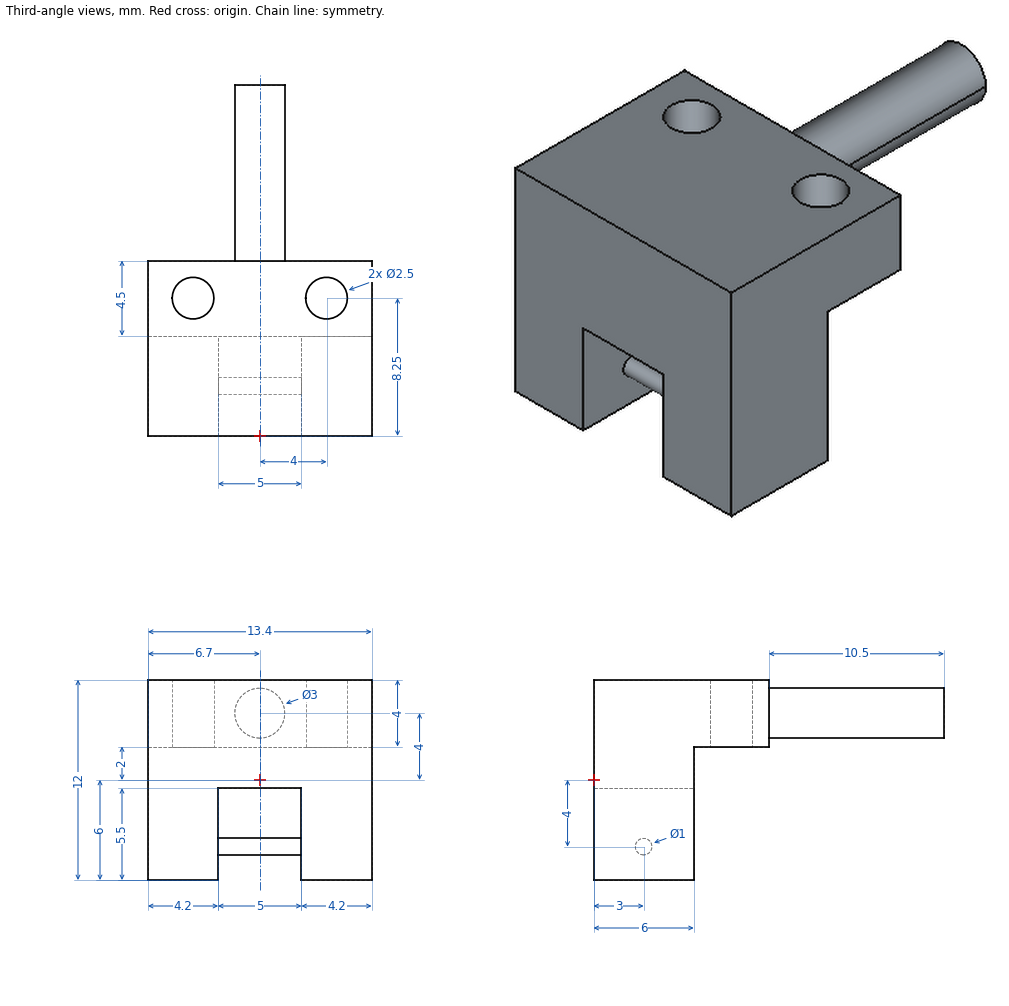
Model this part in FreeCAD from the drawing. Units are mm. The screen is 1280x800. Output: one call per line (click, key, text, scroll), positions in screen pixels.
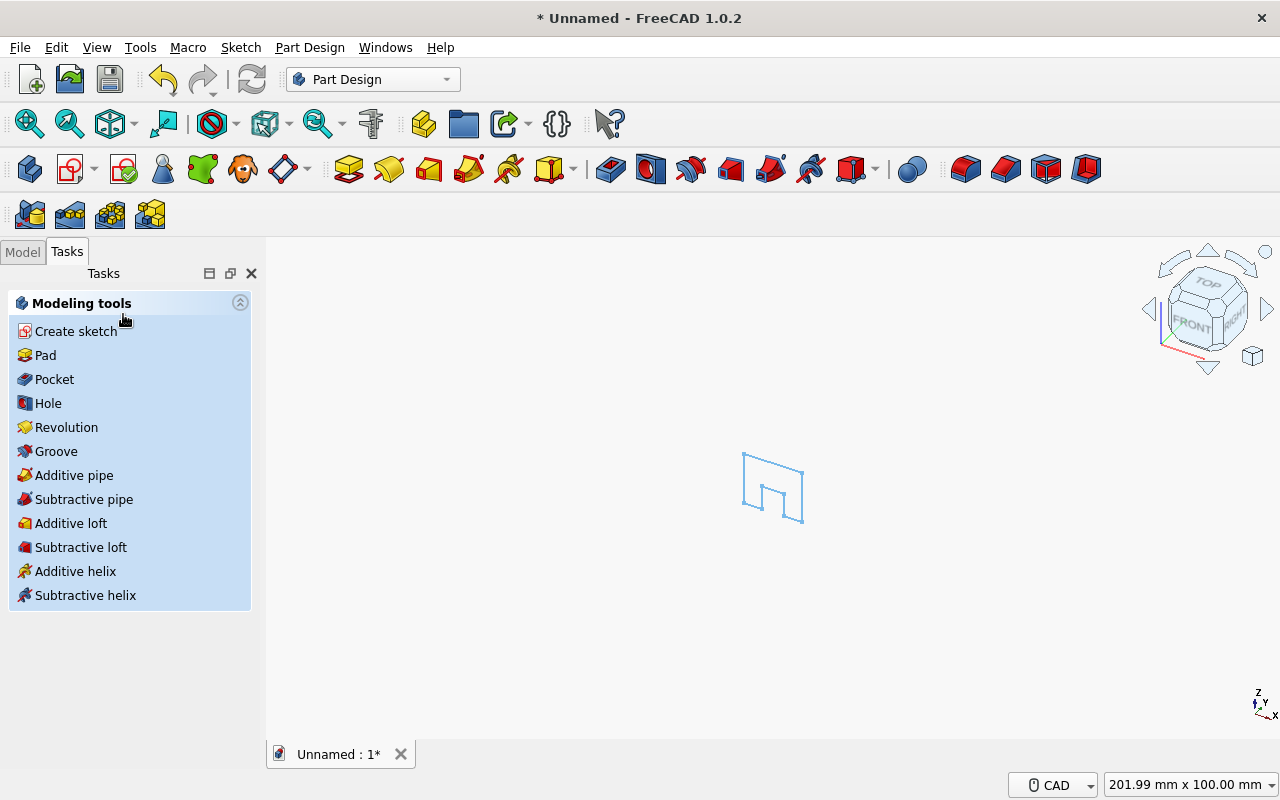
click(350, 170)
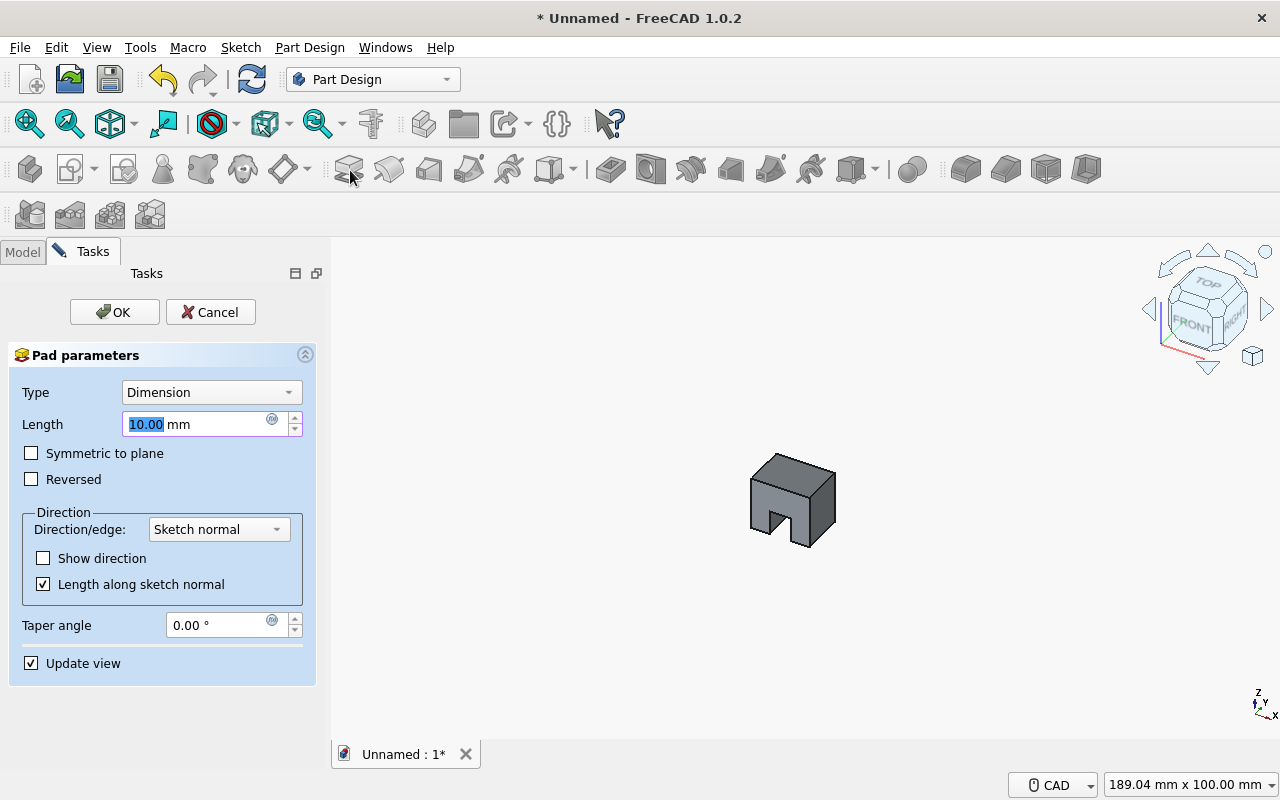
text(6)
key(Tab)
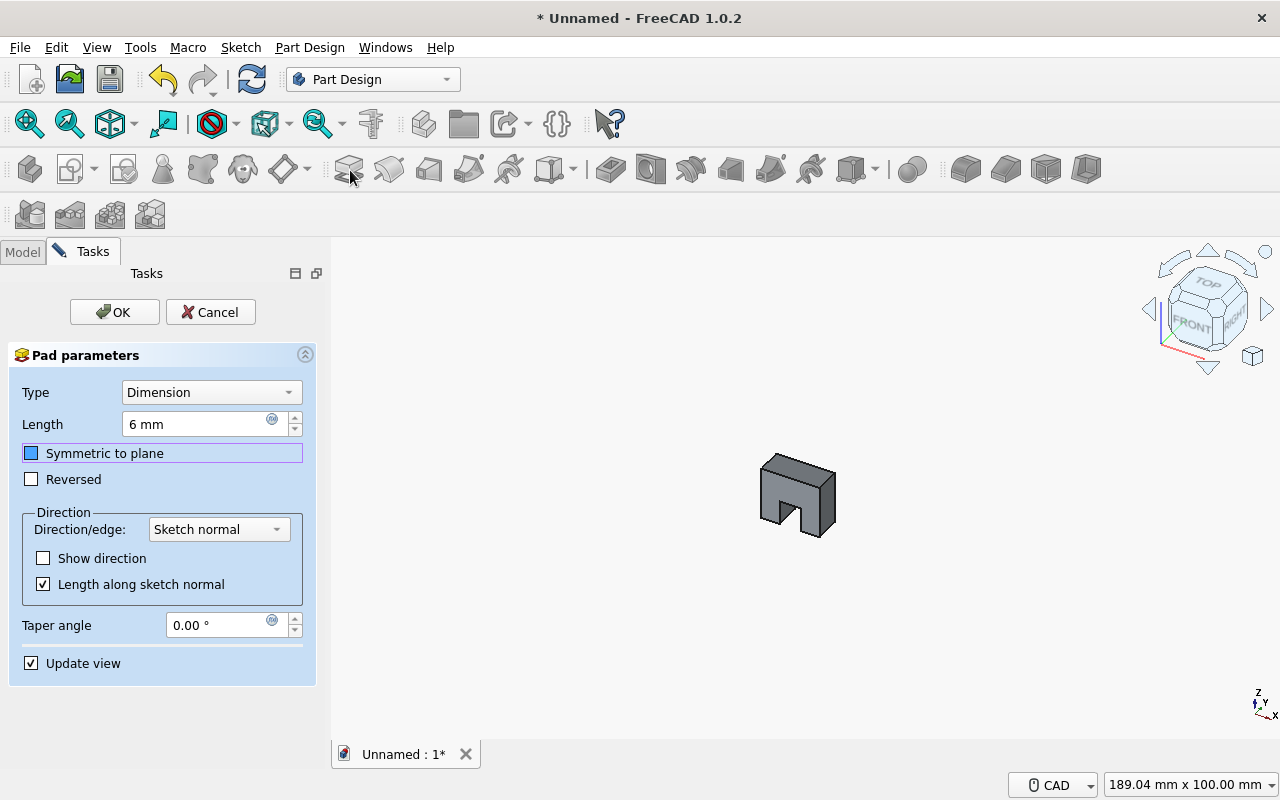
click(30, 479)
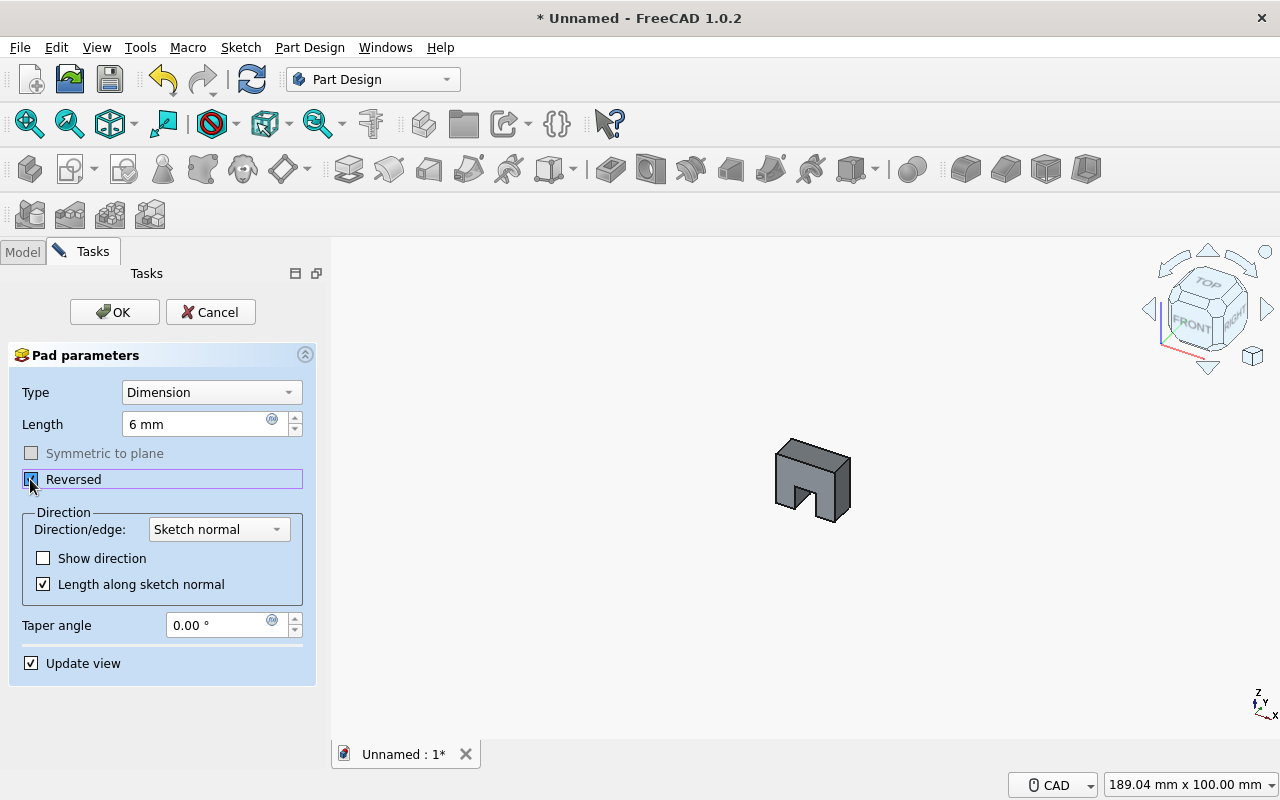
click(115, 312)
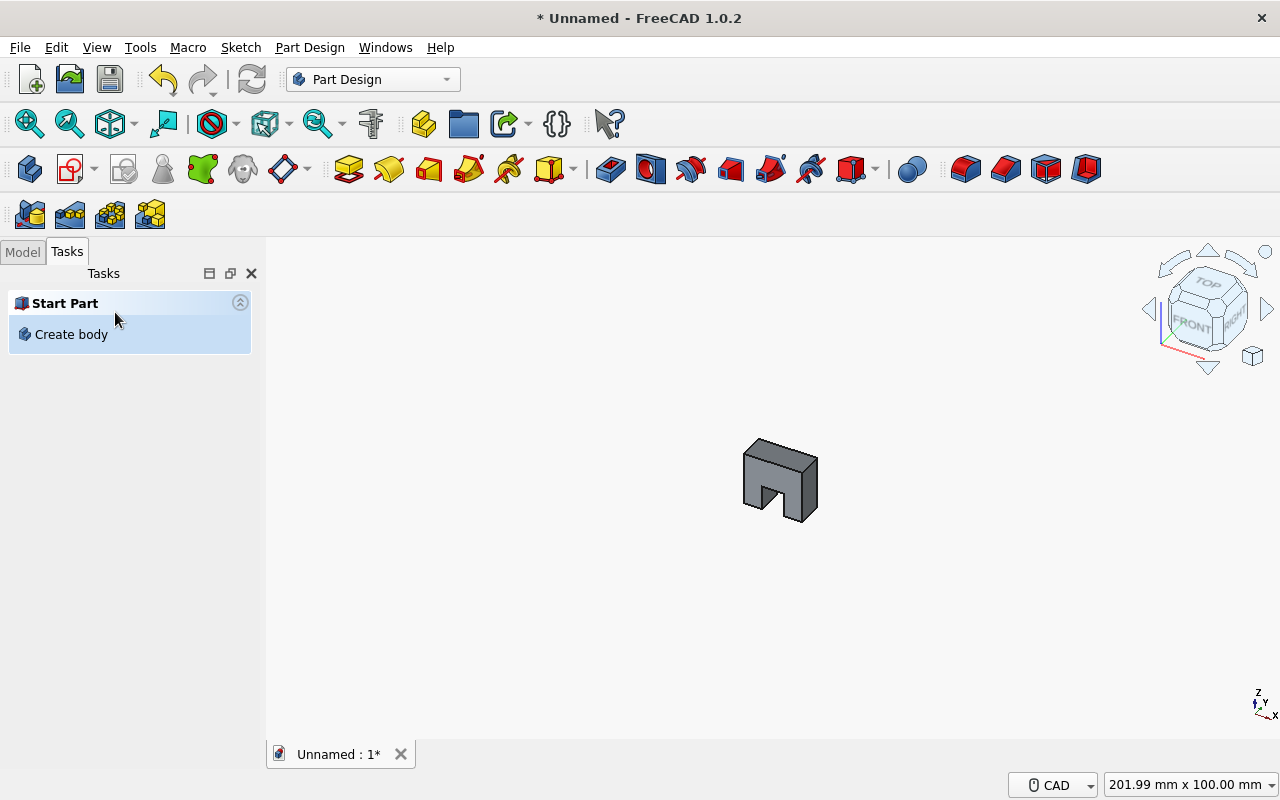
click(30, 124)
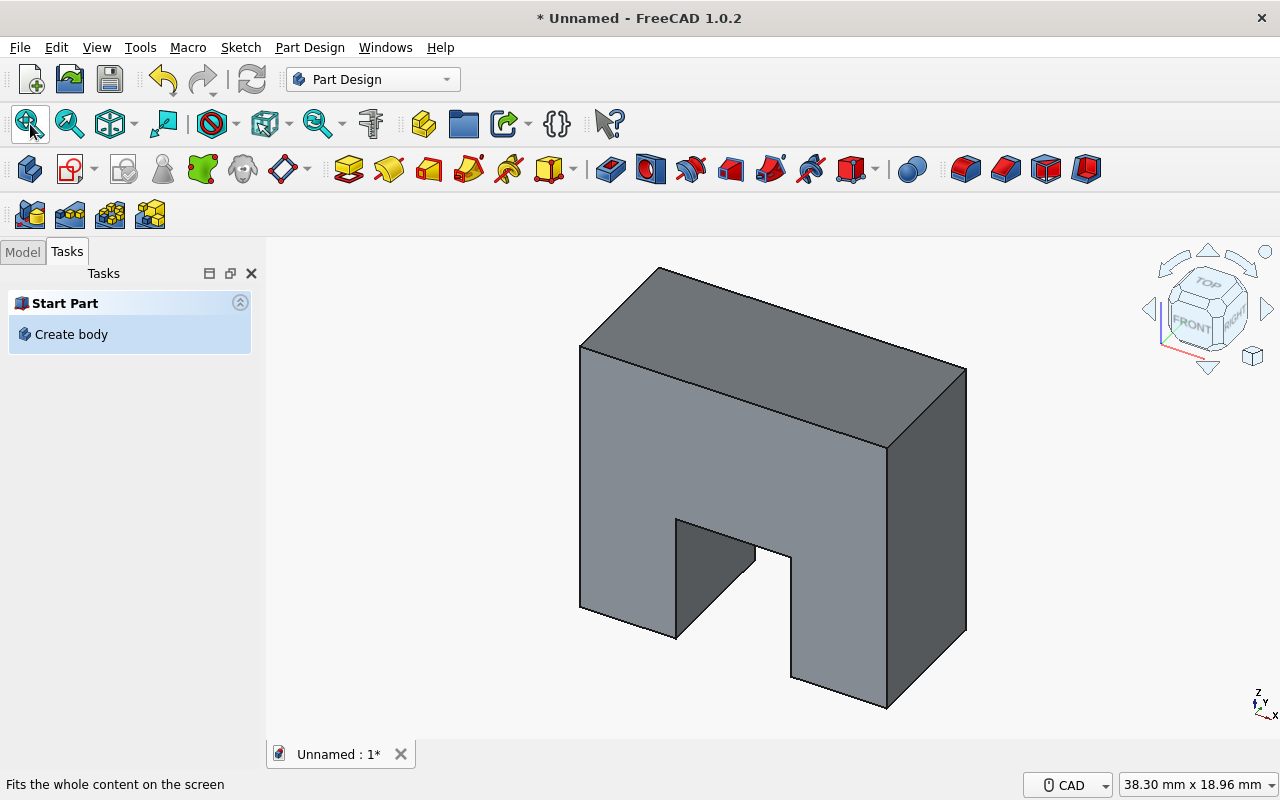
key(4)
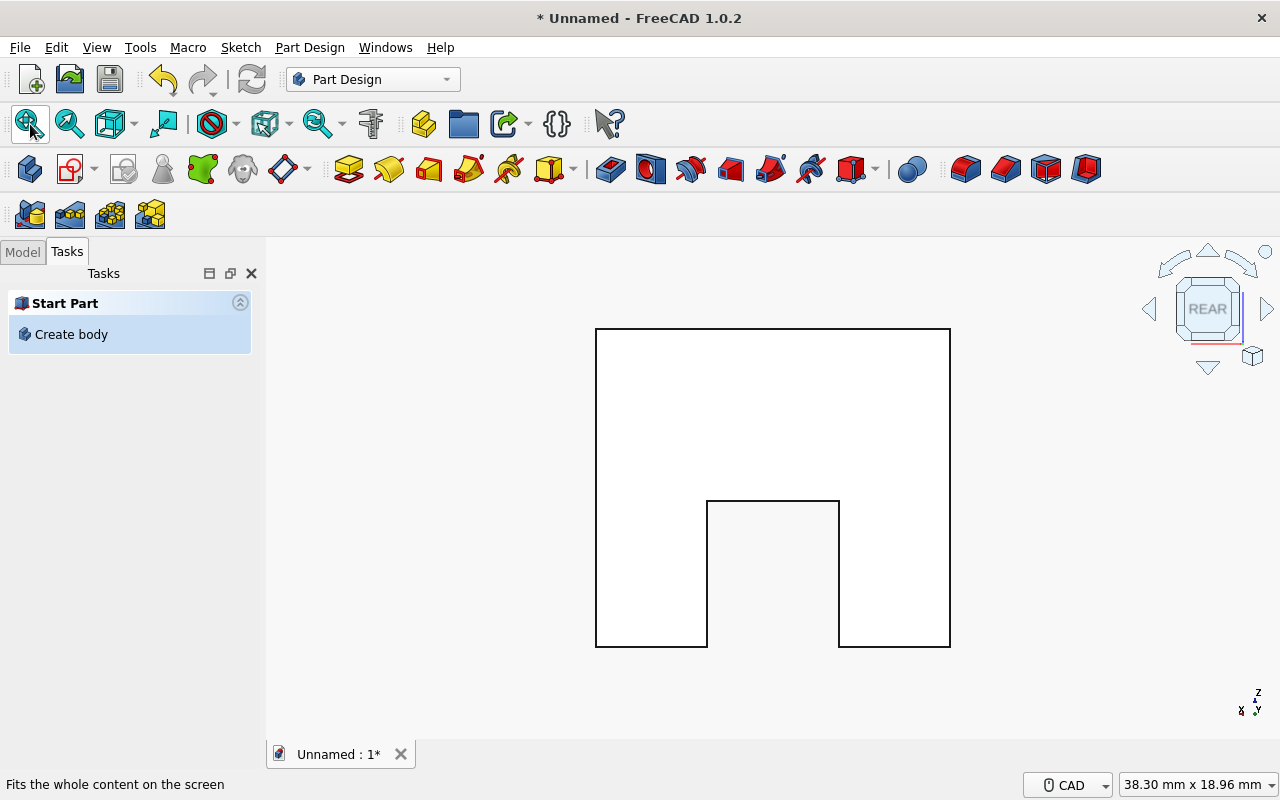
click(874, 442)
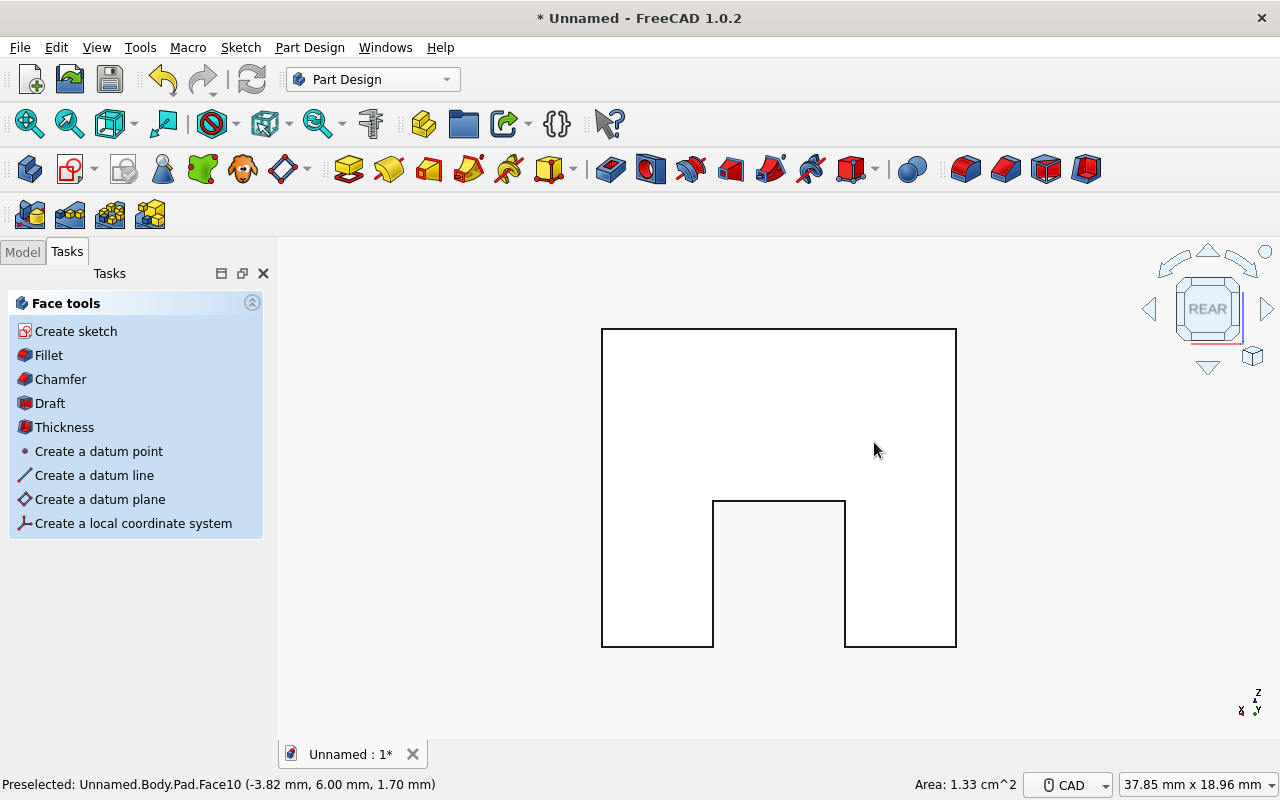
click(70, 170)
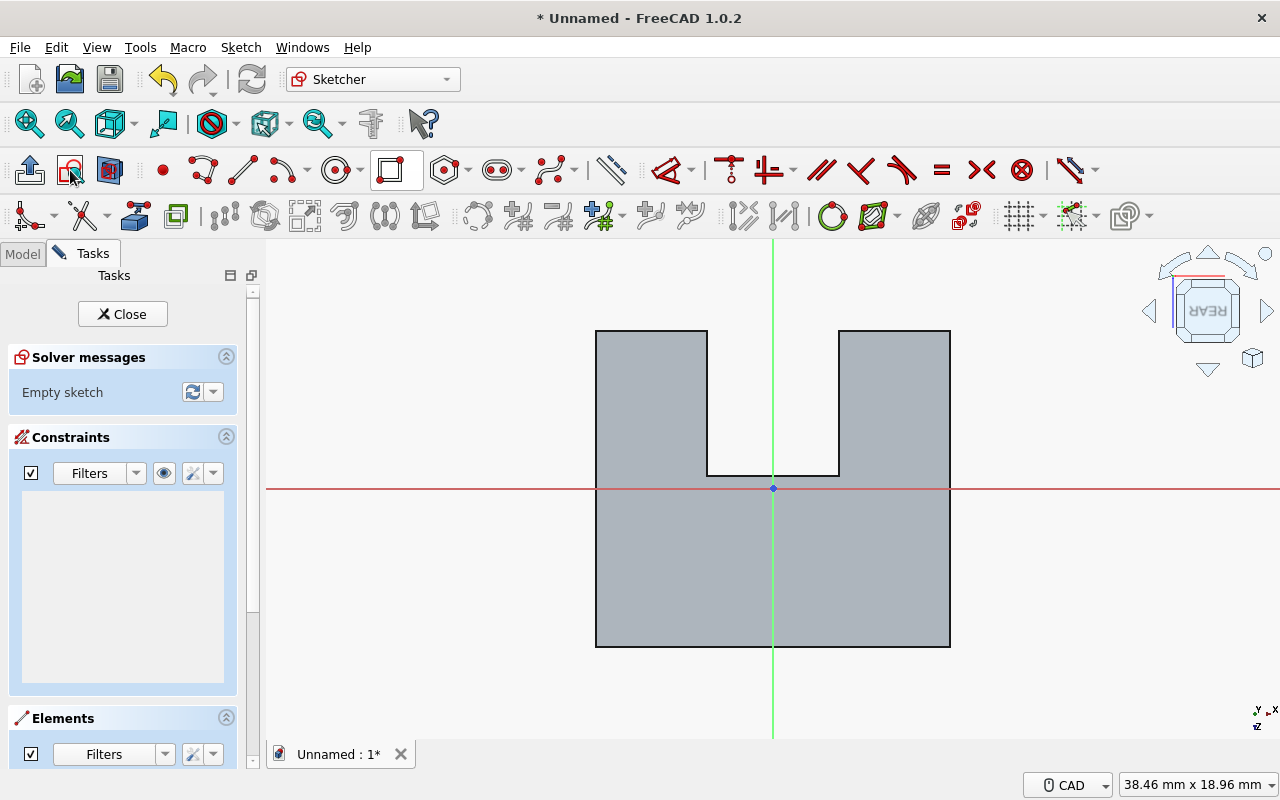
scroll(912, 711, up, 2)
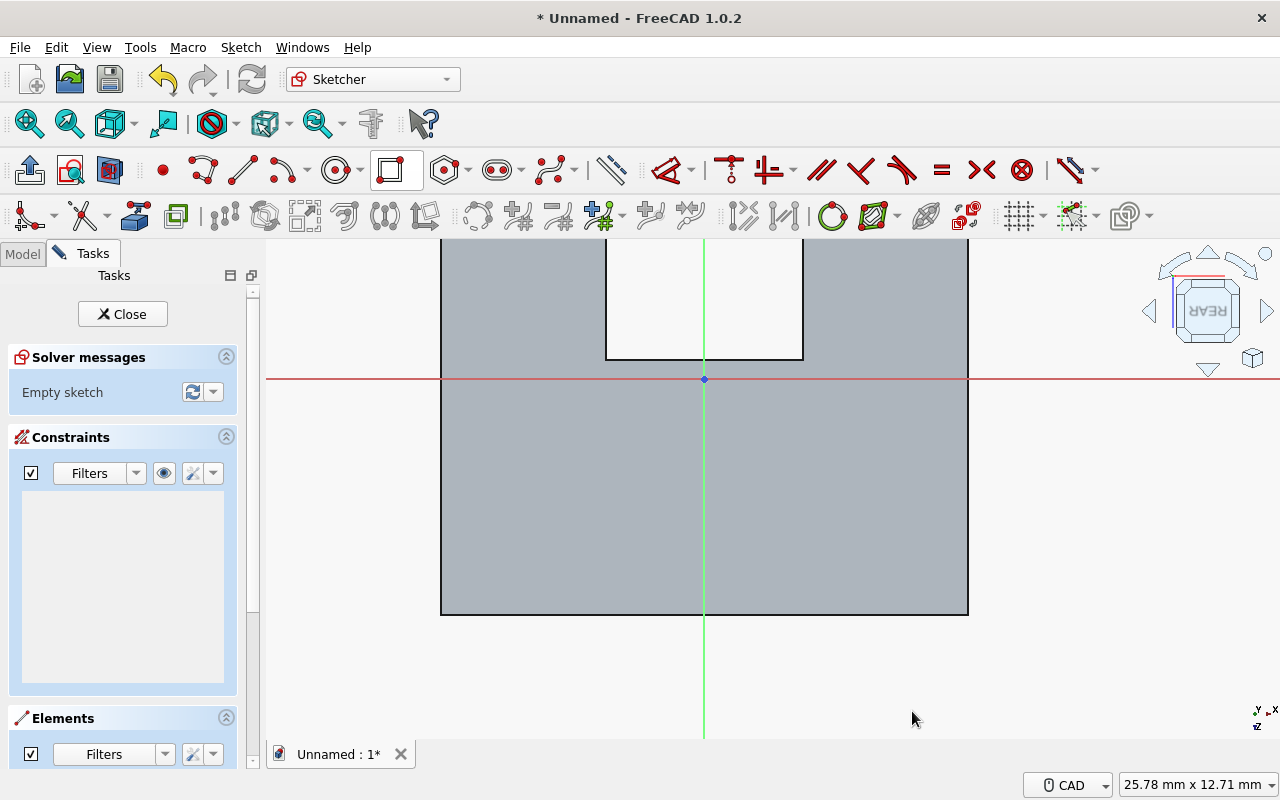
click(390, 170)